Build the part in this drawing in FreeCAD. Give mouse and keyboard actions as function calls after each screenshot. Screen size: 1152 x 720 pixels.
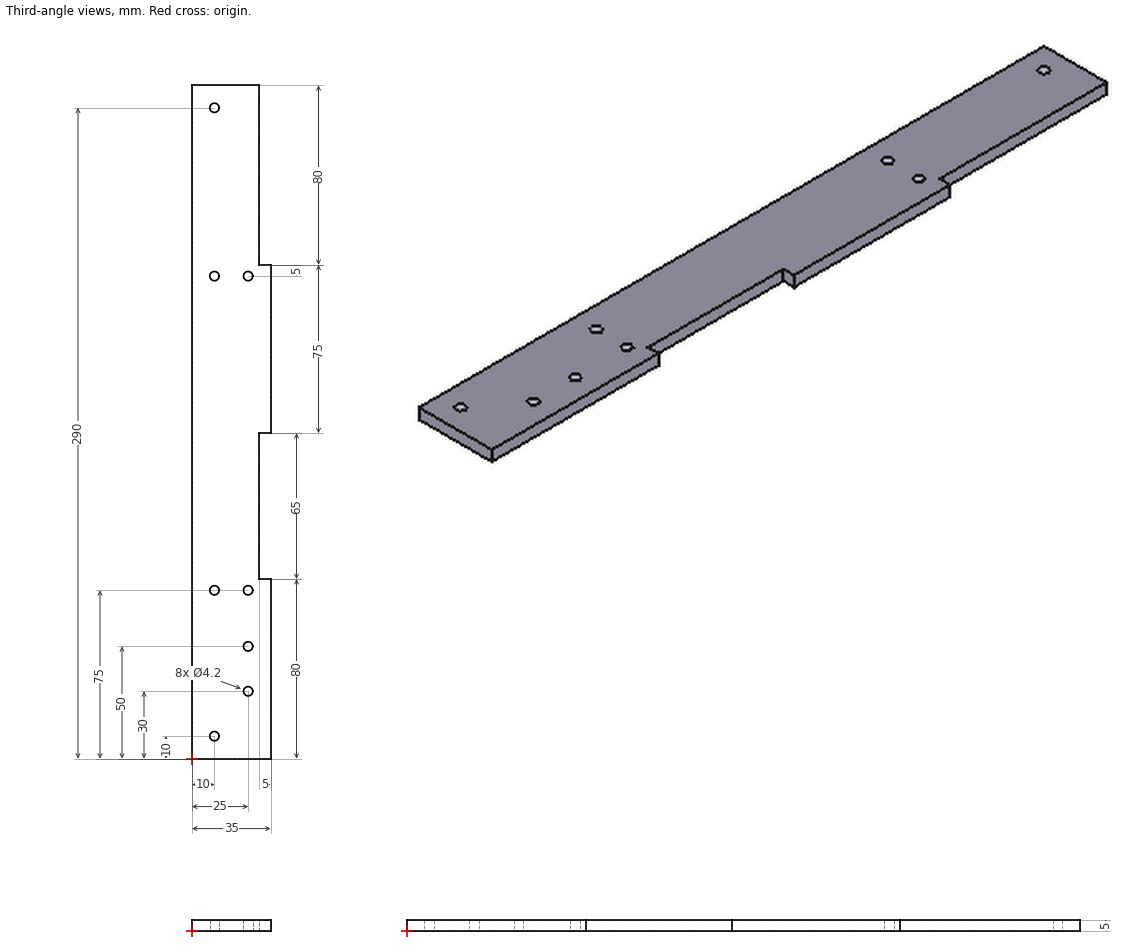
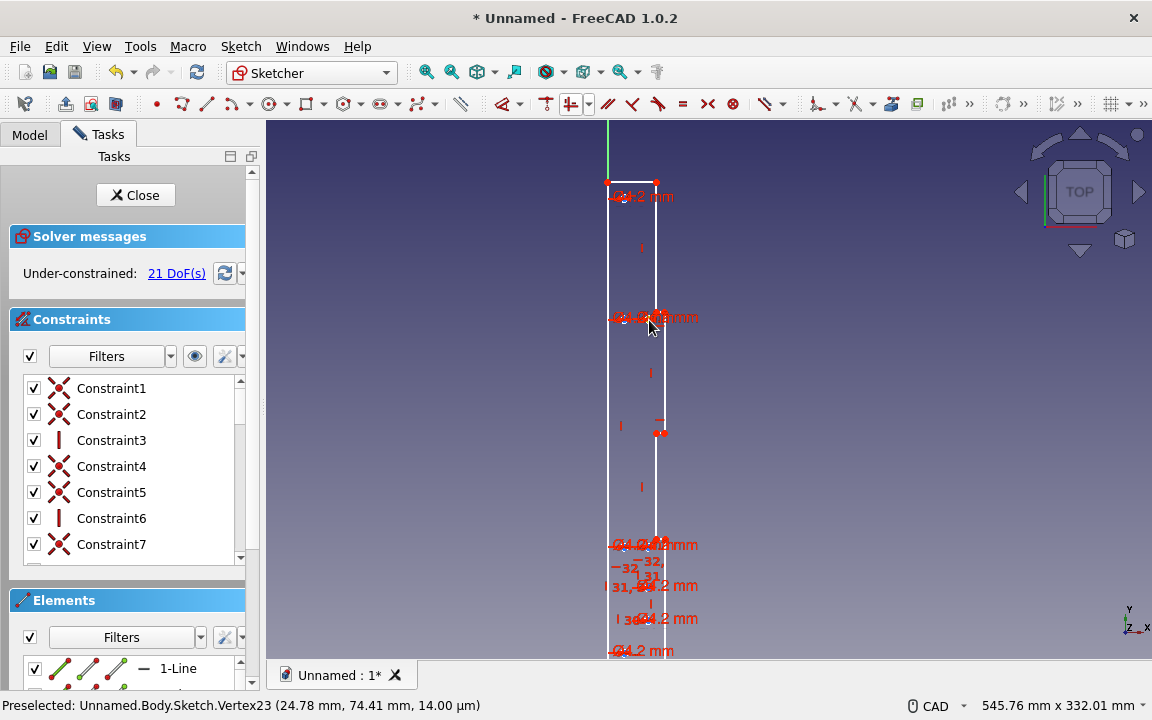
click(648, 319)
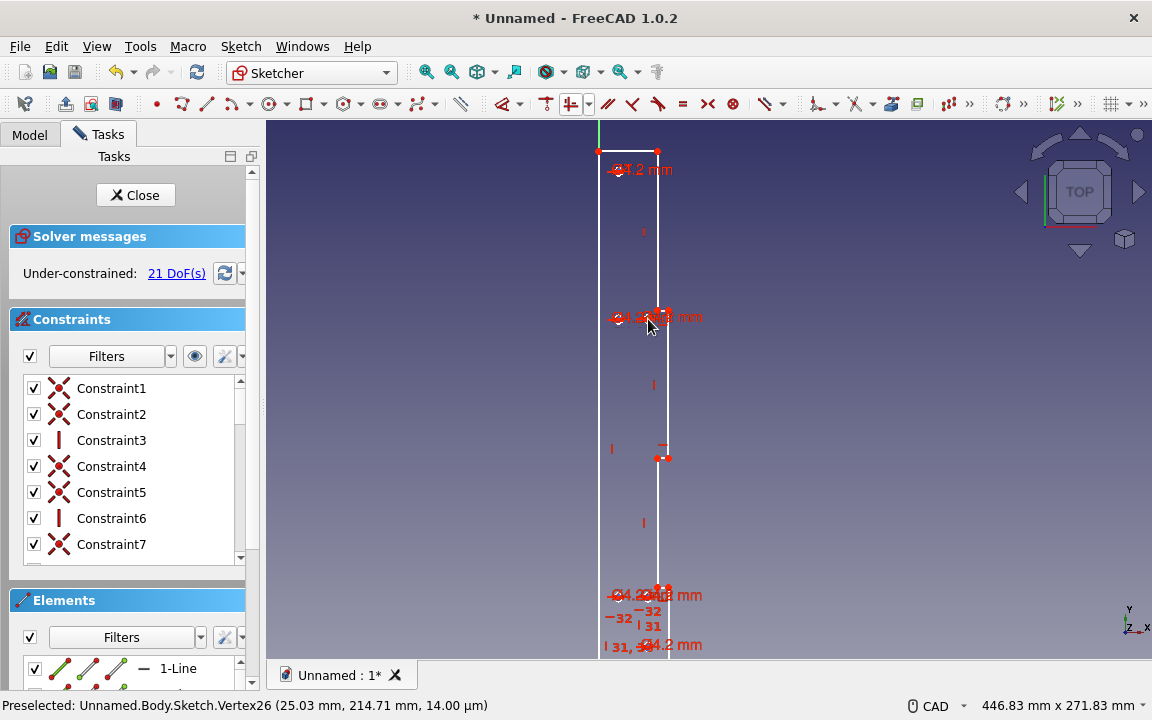
click(619, 320)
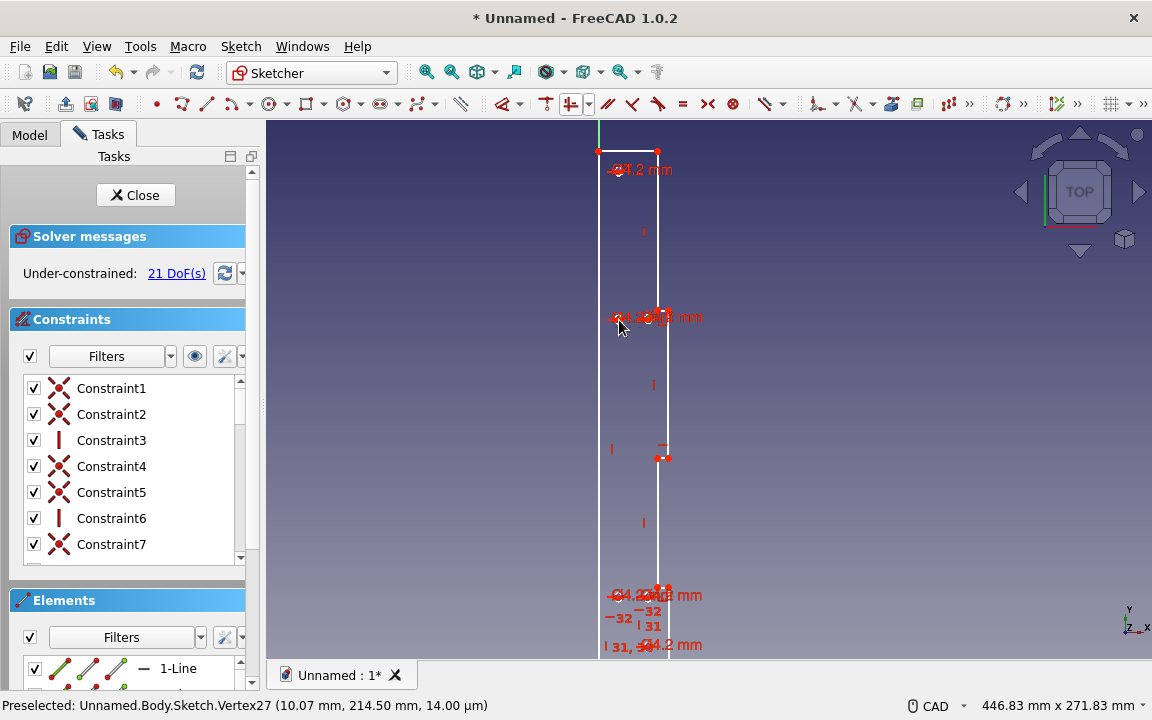
key(h)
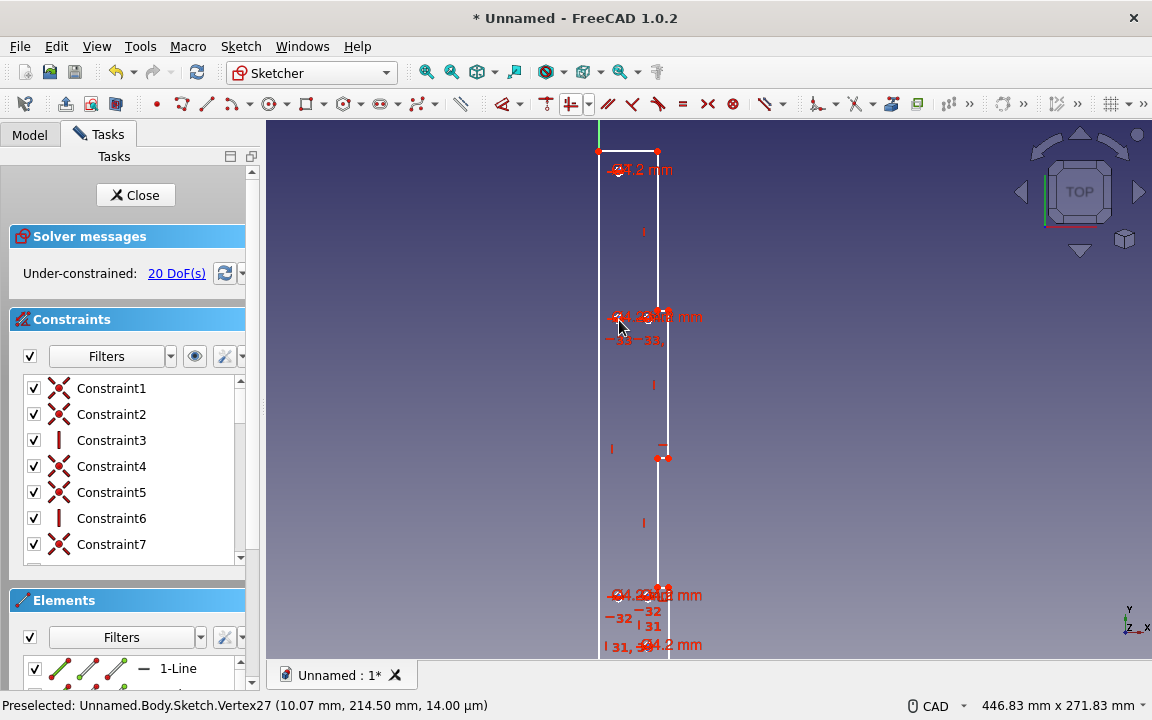
click(502, 104)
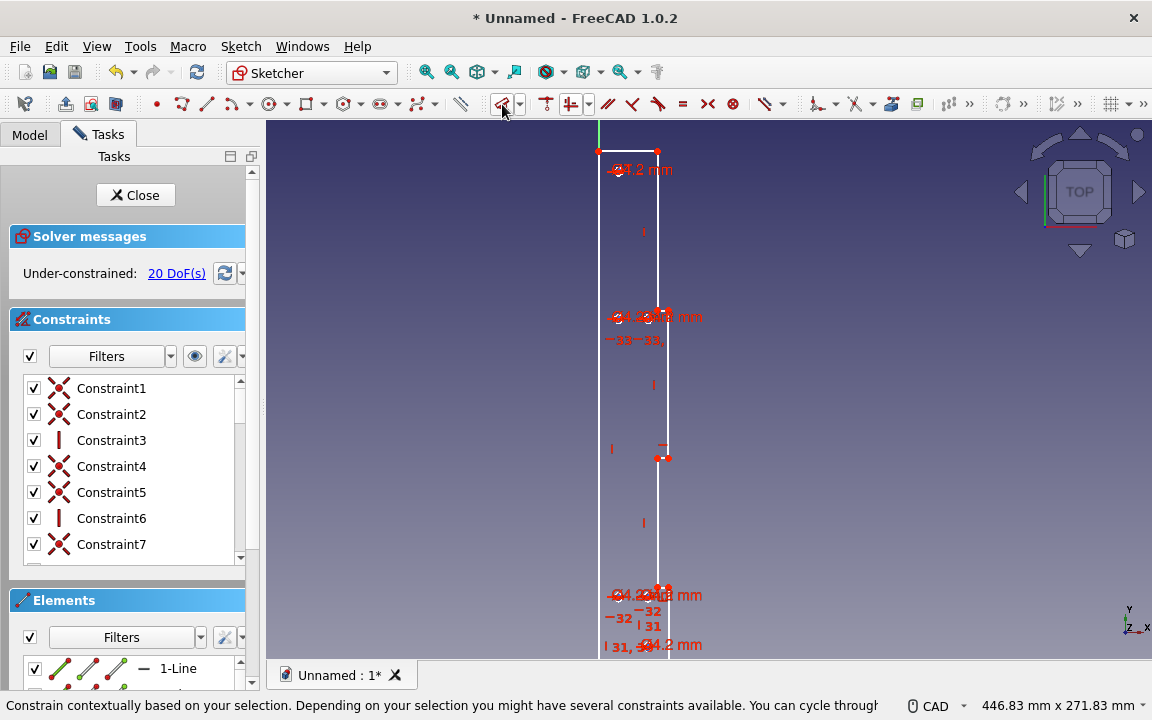
scroll(663, 588, up, 7)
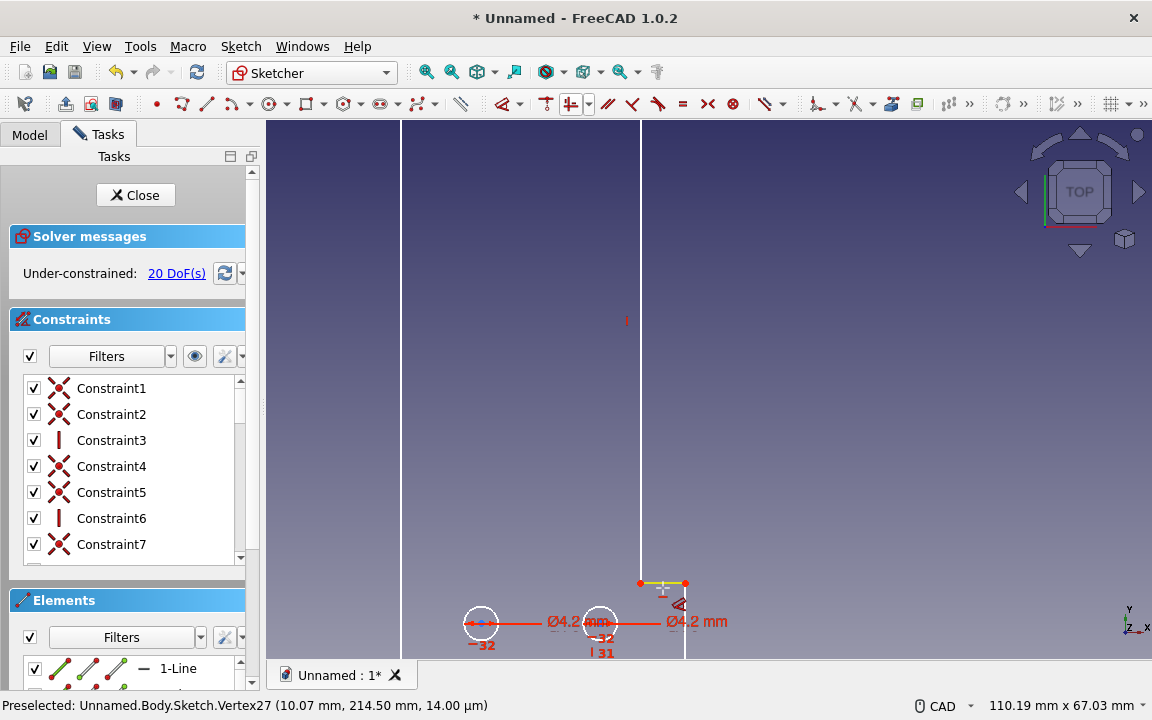
click(663, 583)
click(663, 617)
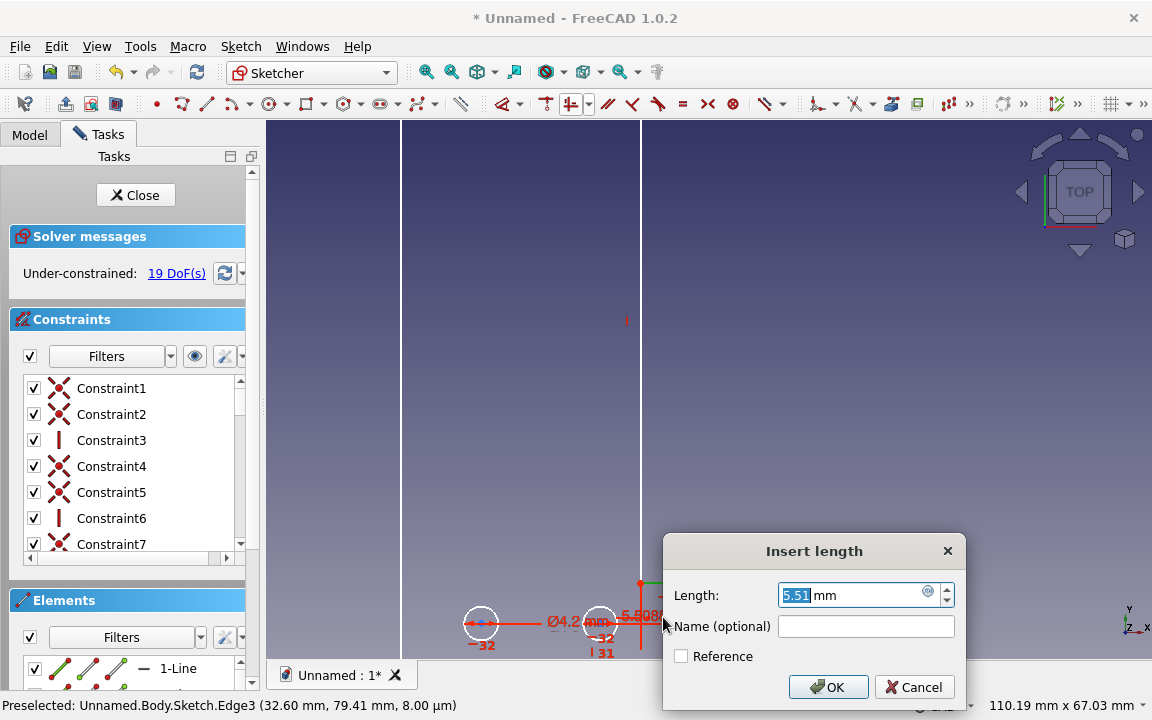
text(5)
key(Return)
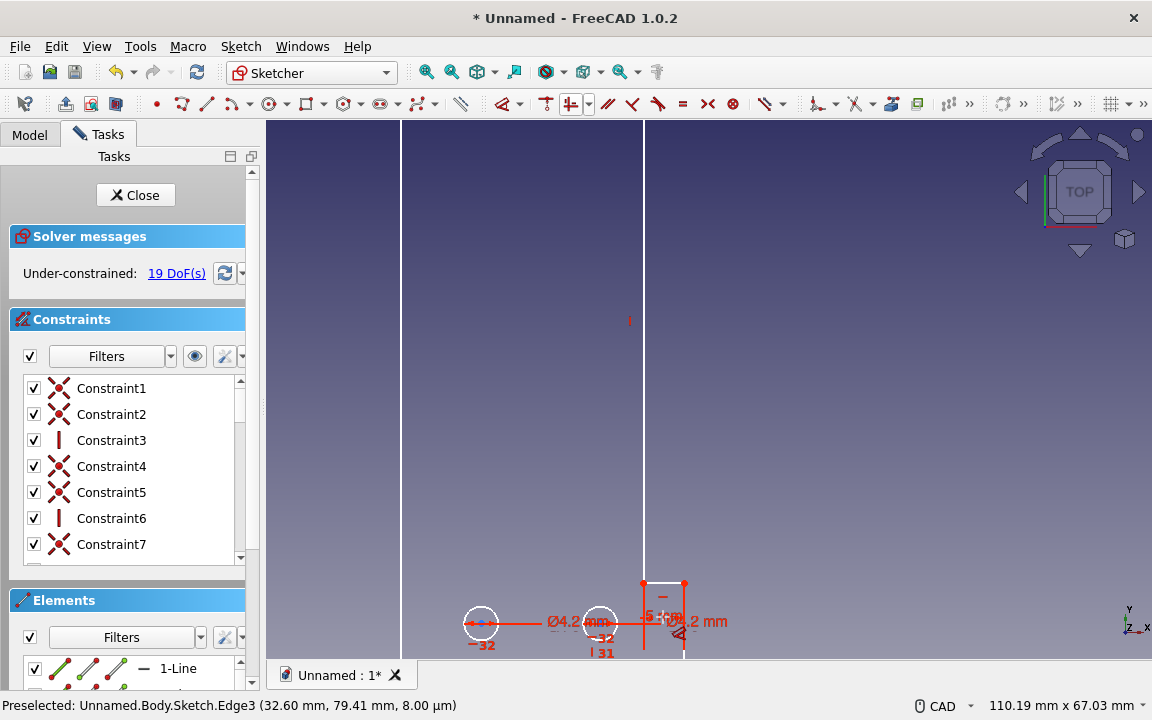
scroll(656, 448, down, 10)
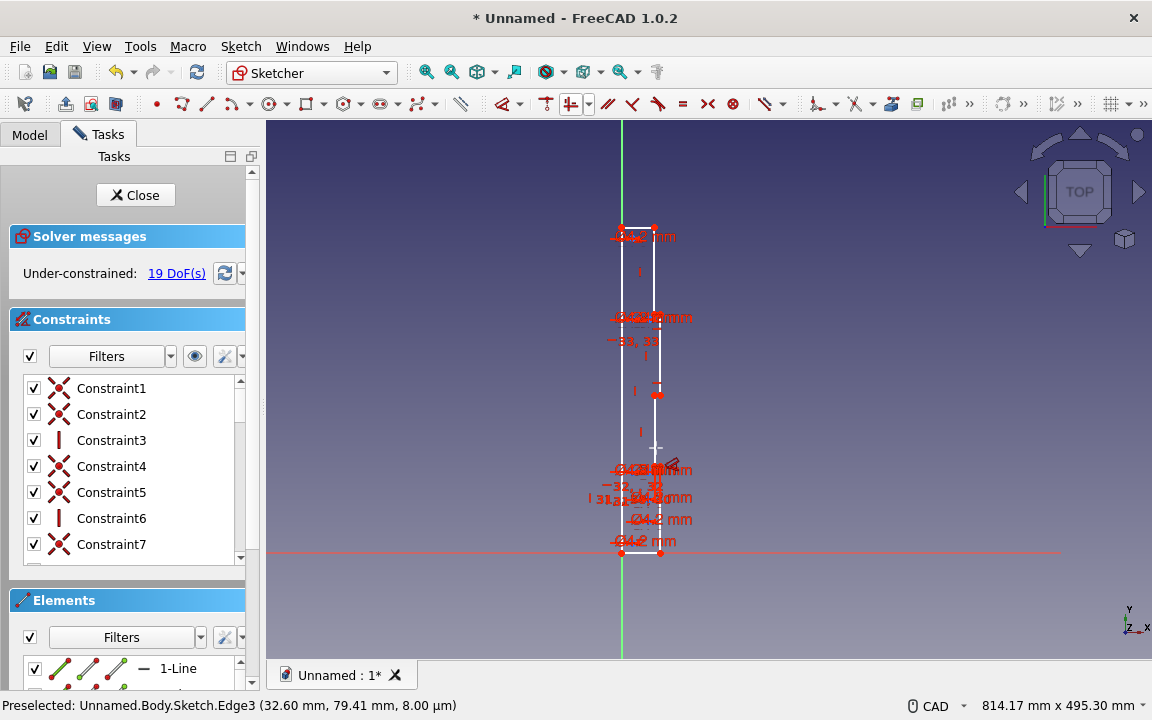
scroll(656, 396, up, 11)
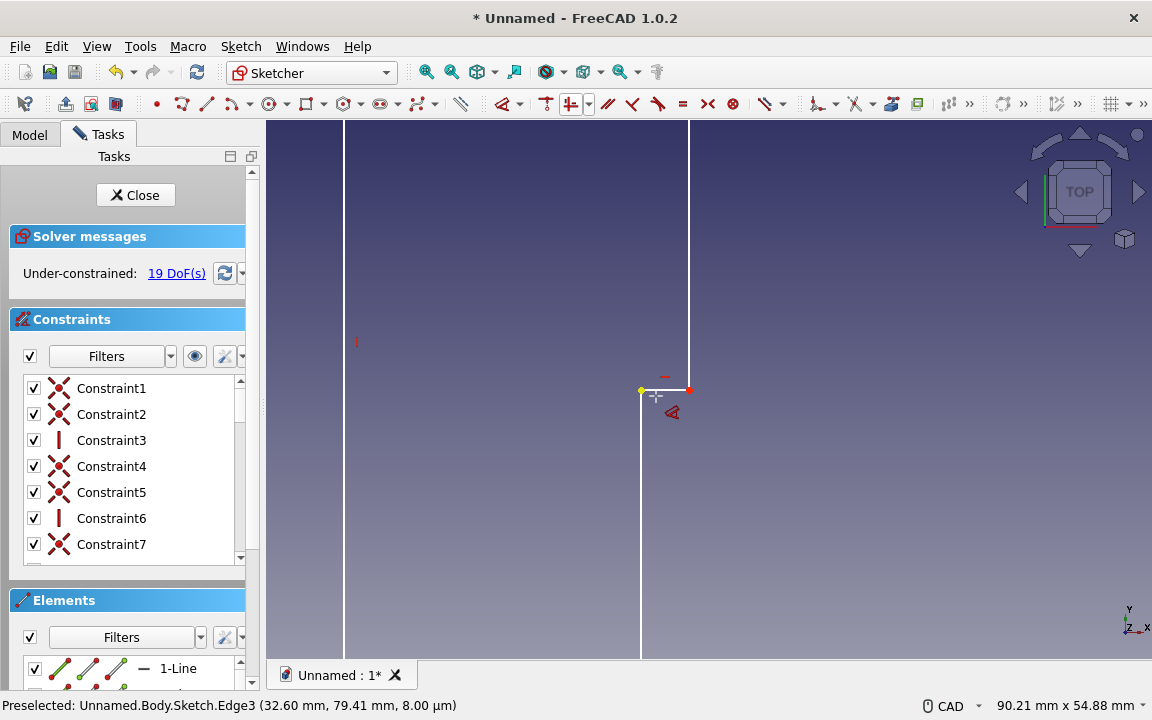
click(656, 390)
click(665, 424)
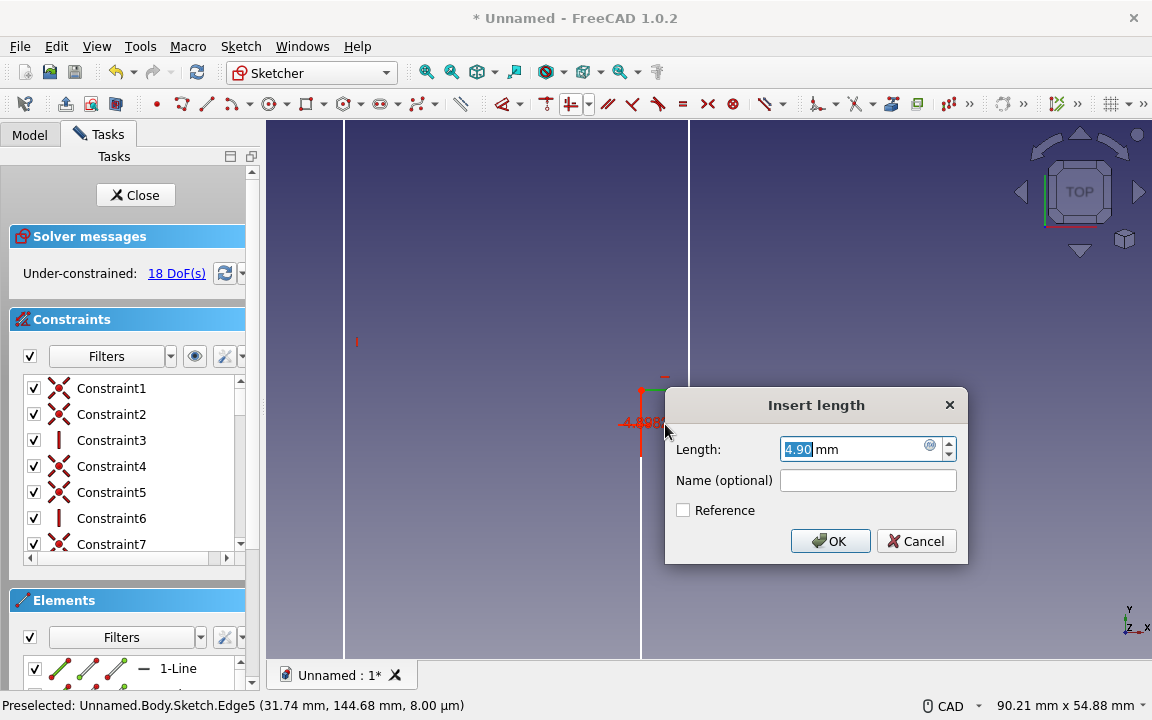
text(5)
key(Return)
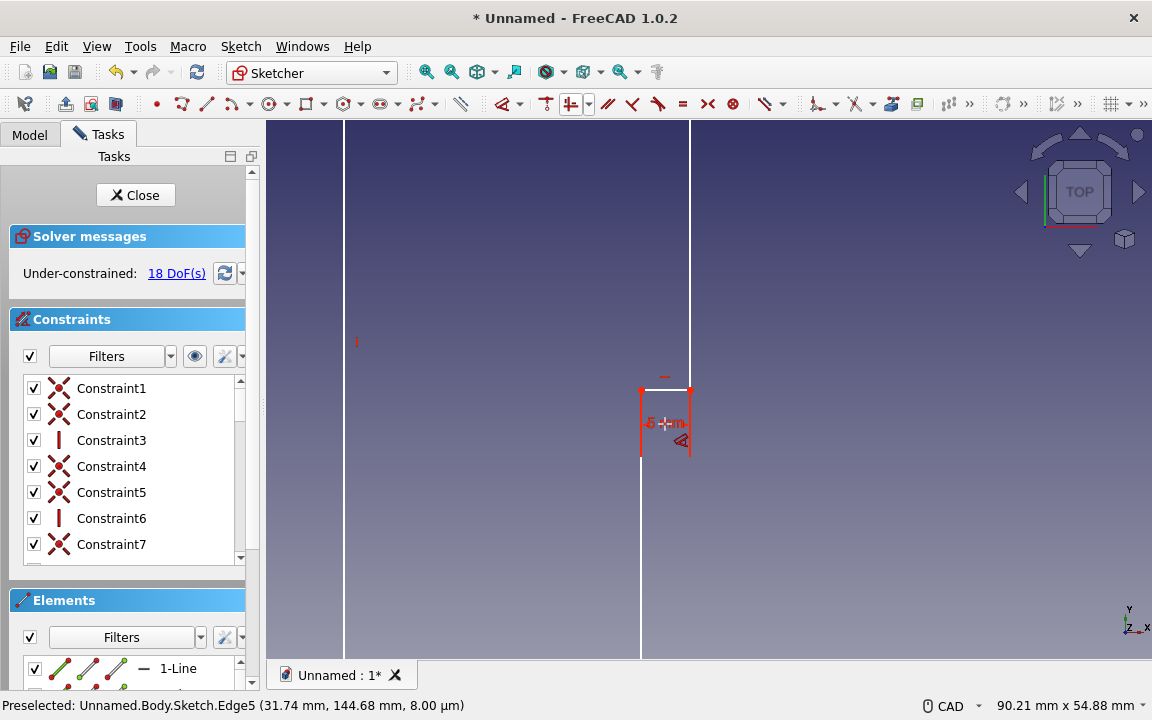
scroll(656, 396, down, 11)